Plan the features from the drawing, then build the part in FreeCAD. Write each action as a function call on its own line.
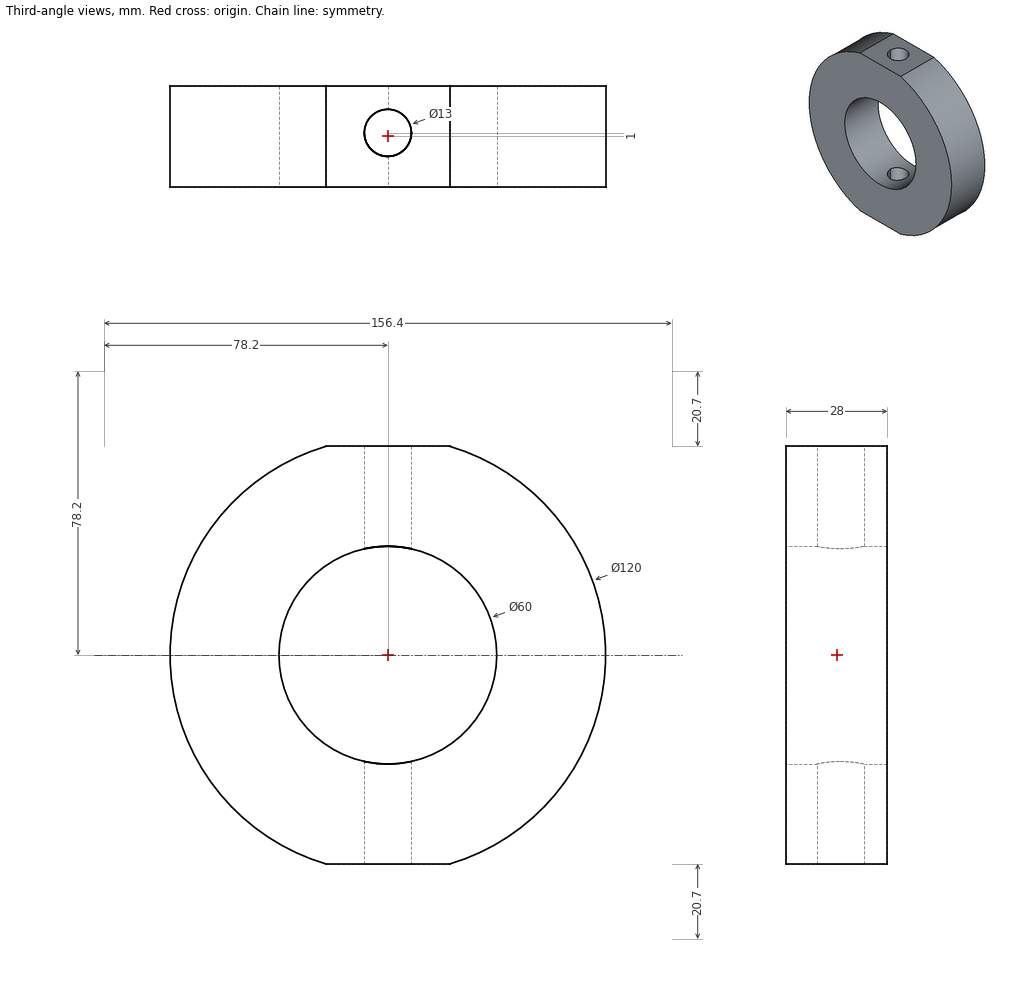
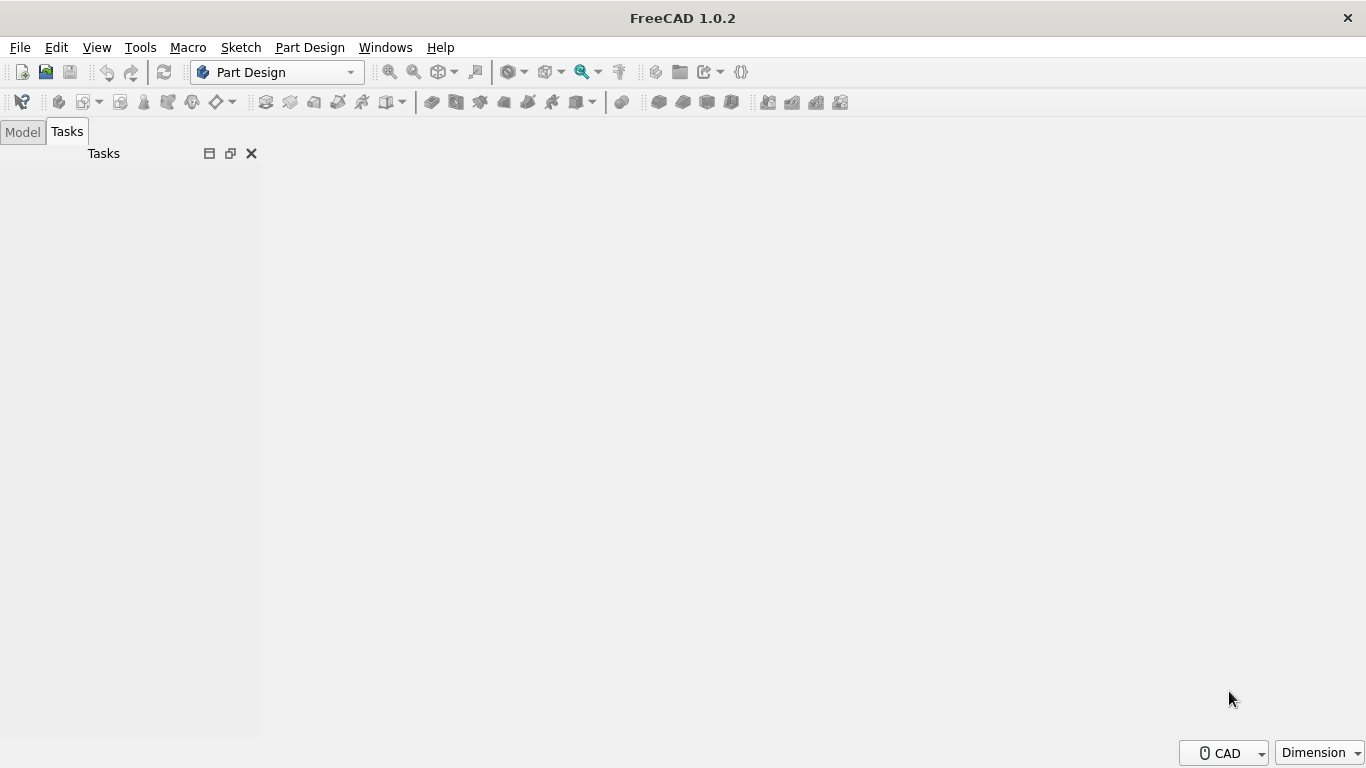
key(ctrl+n)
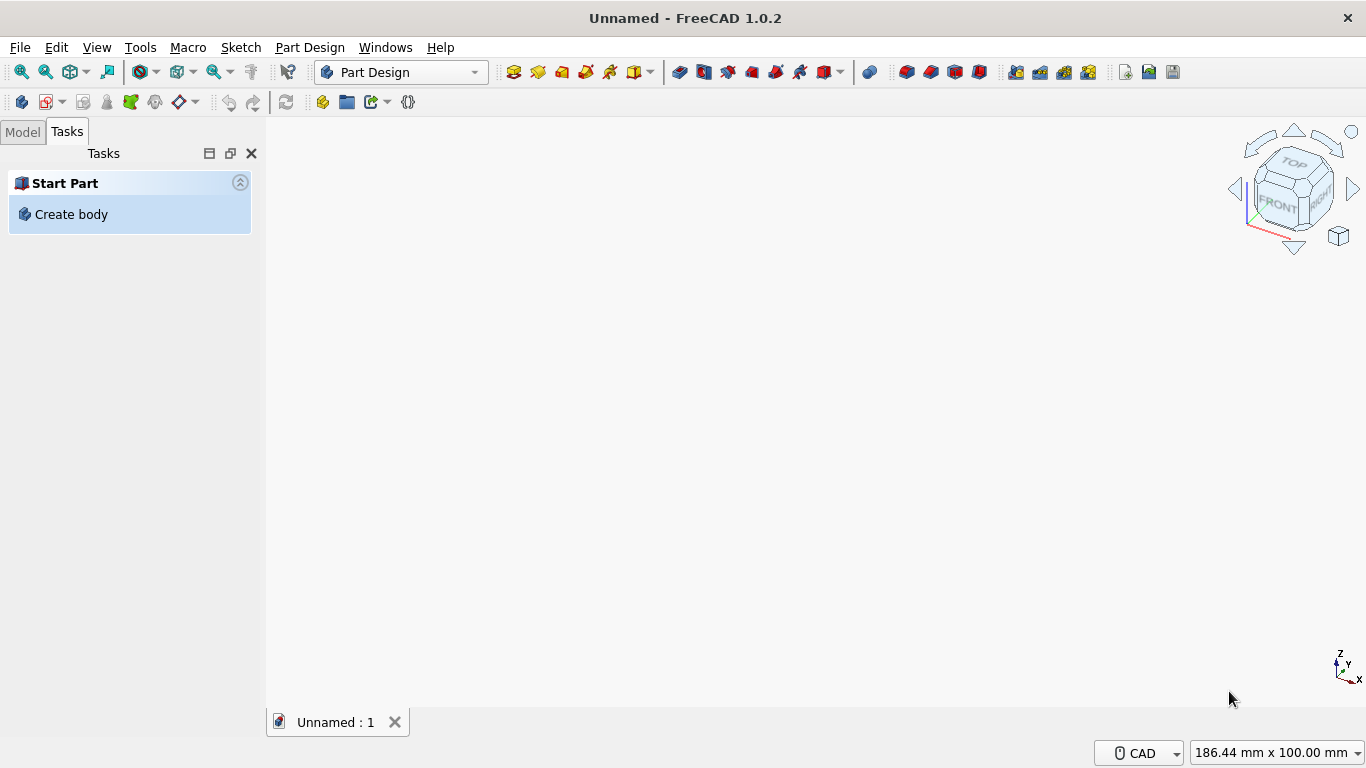
click(46, 102)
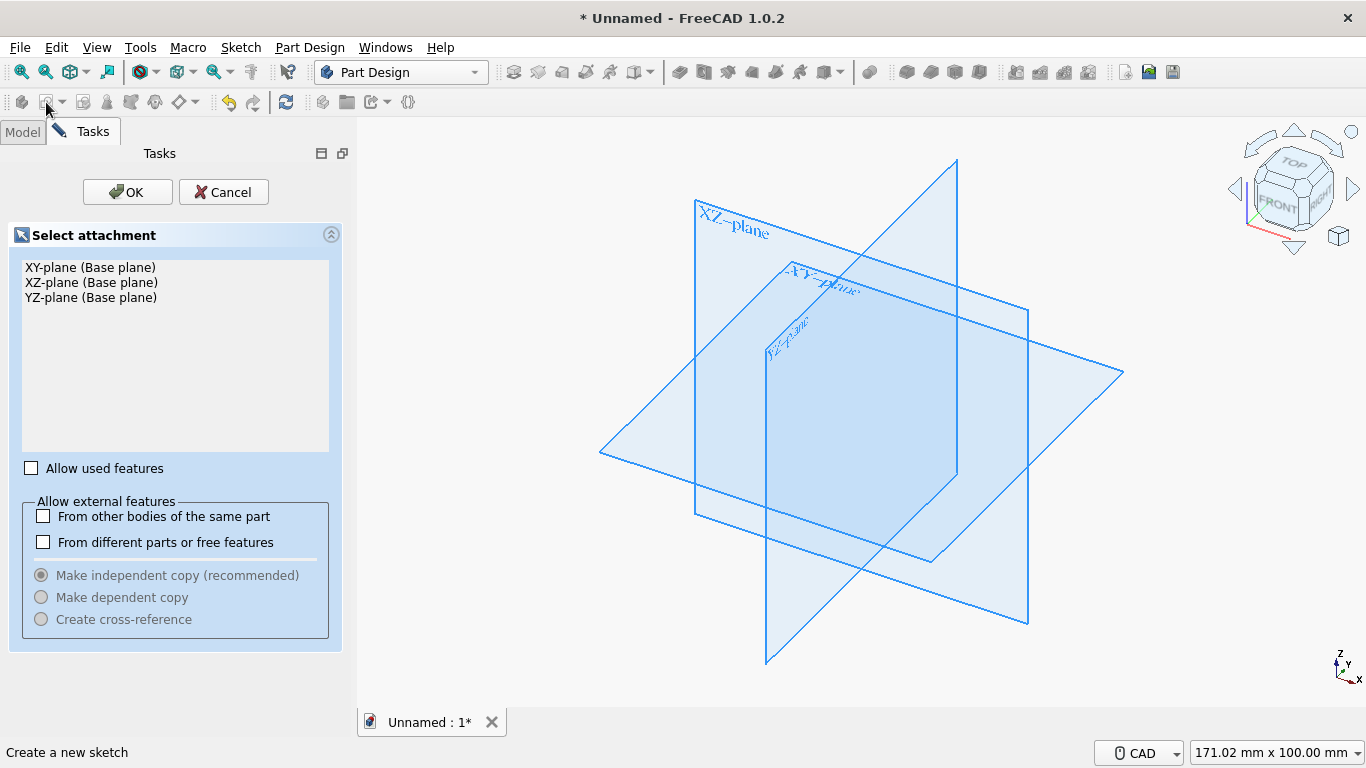
click(82, 282)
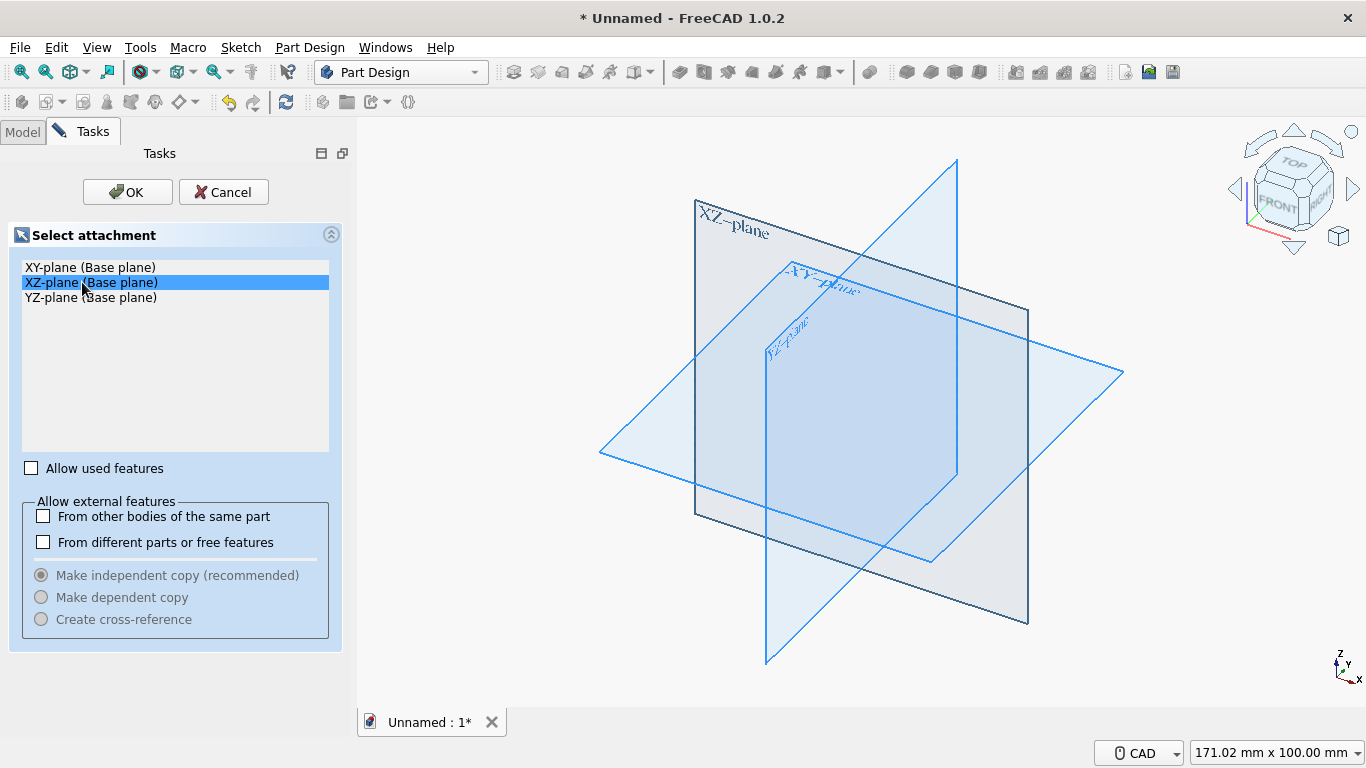
click(128, 192)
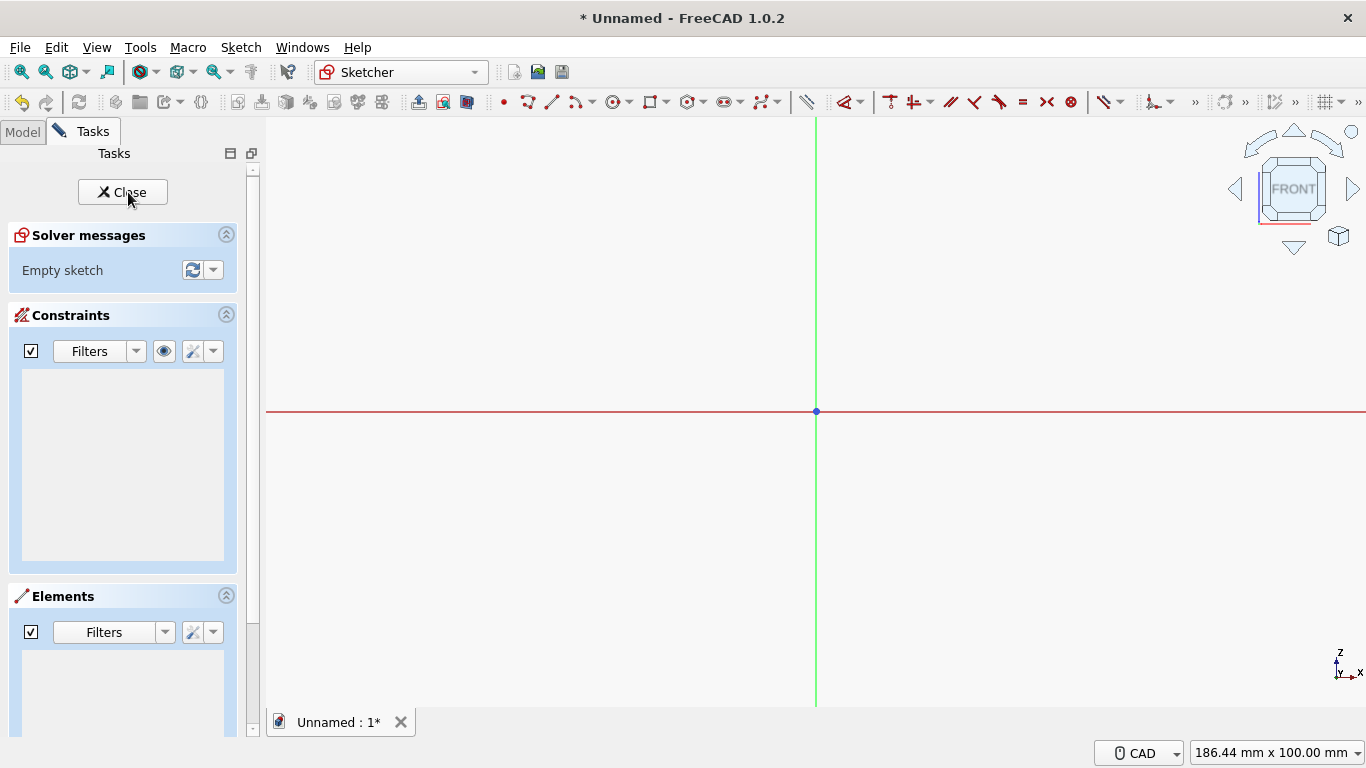
scroll(664, 412, down, 3)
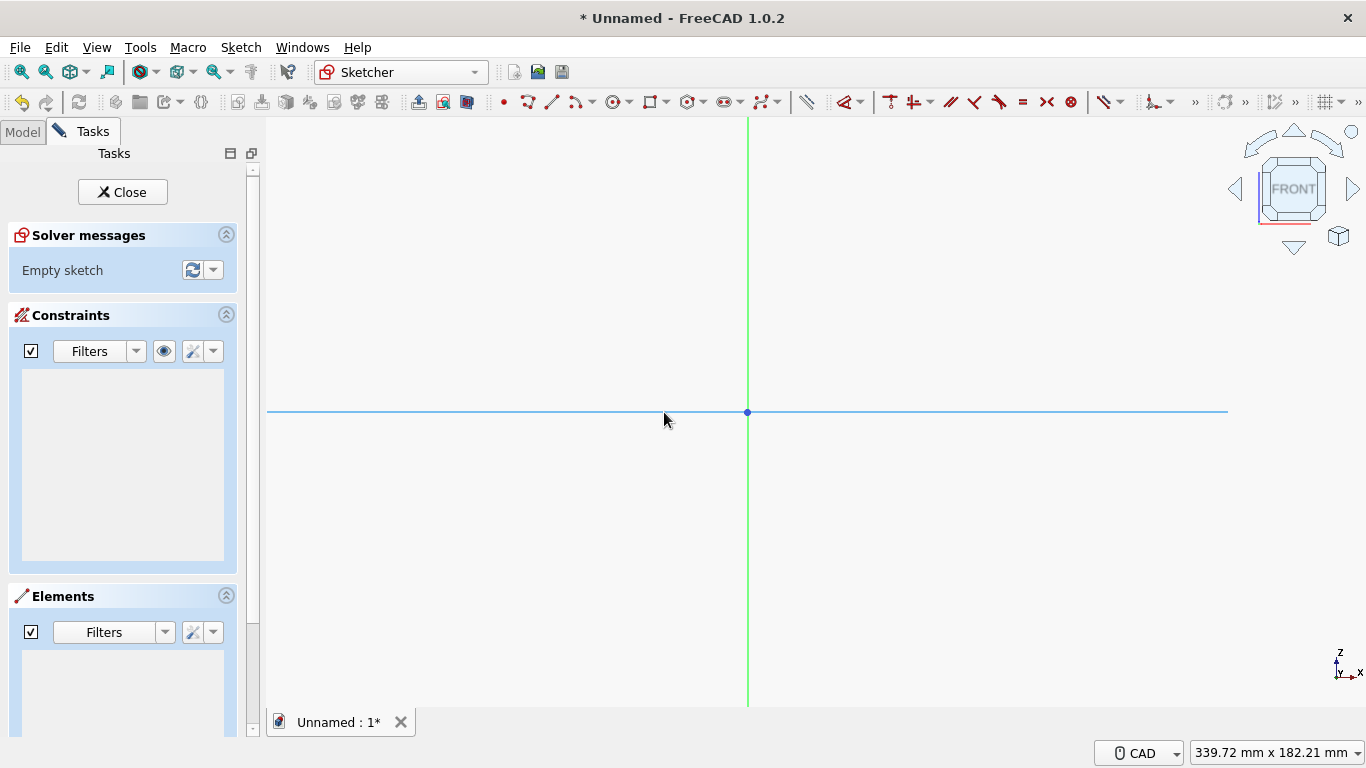
key(g)
key(c)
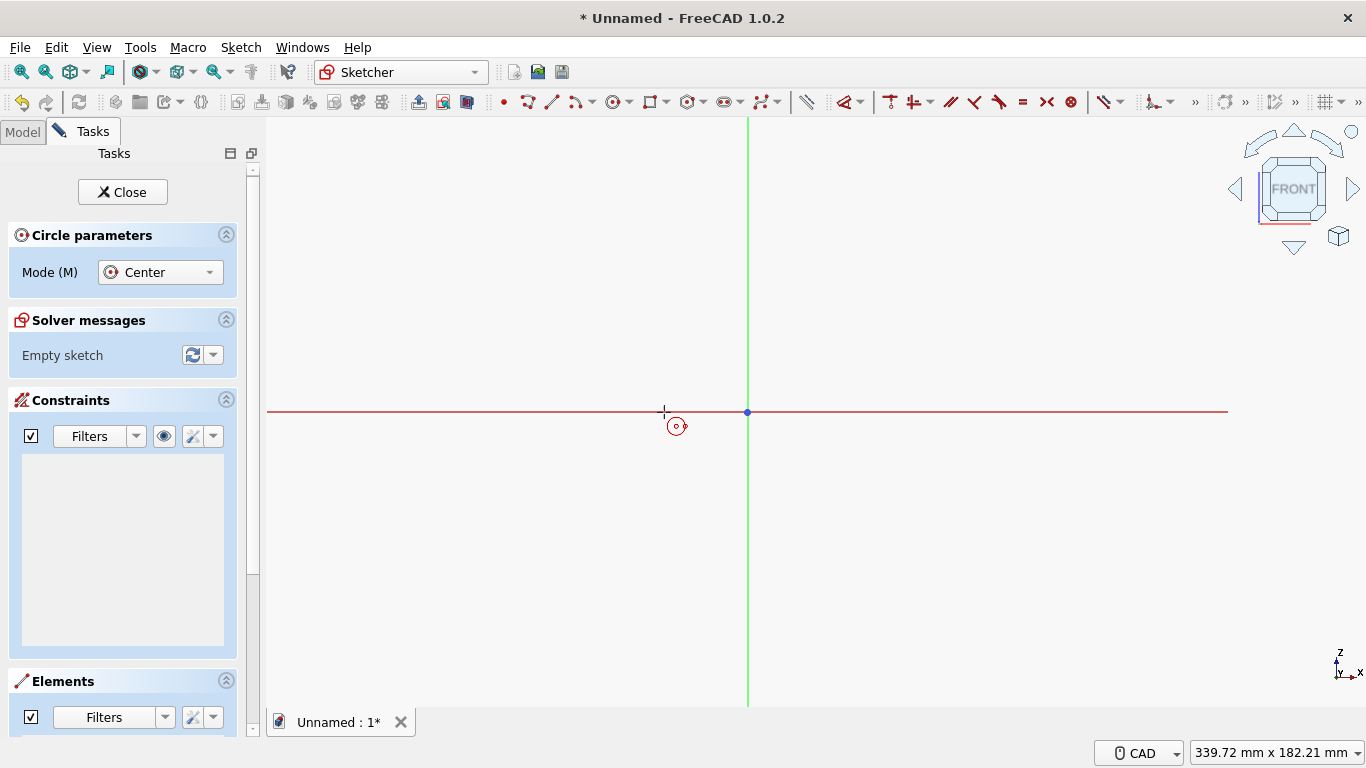
click(748, 412)
move(885, 275)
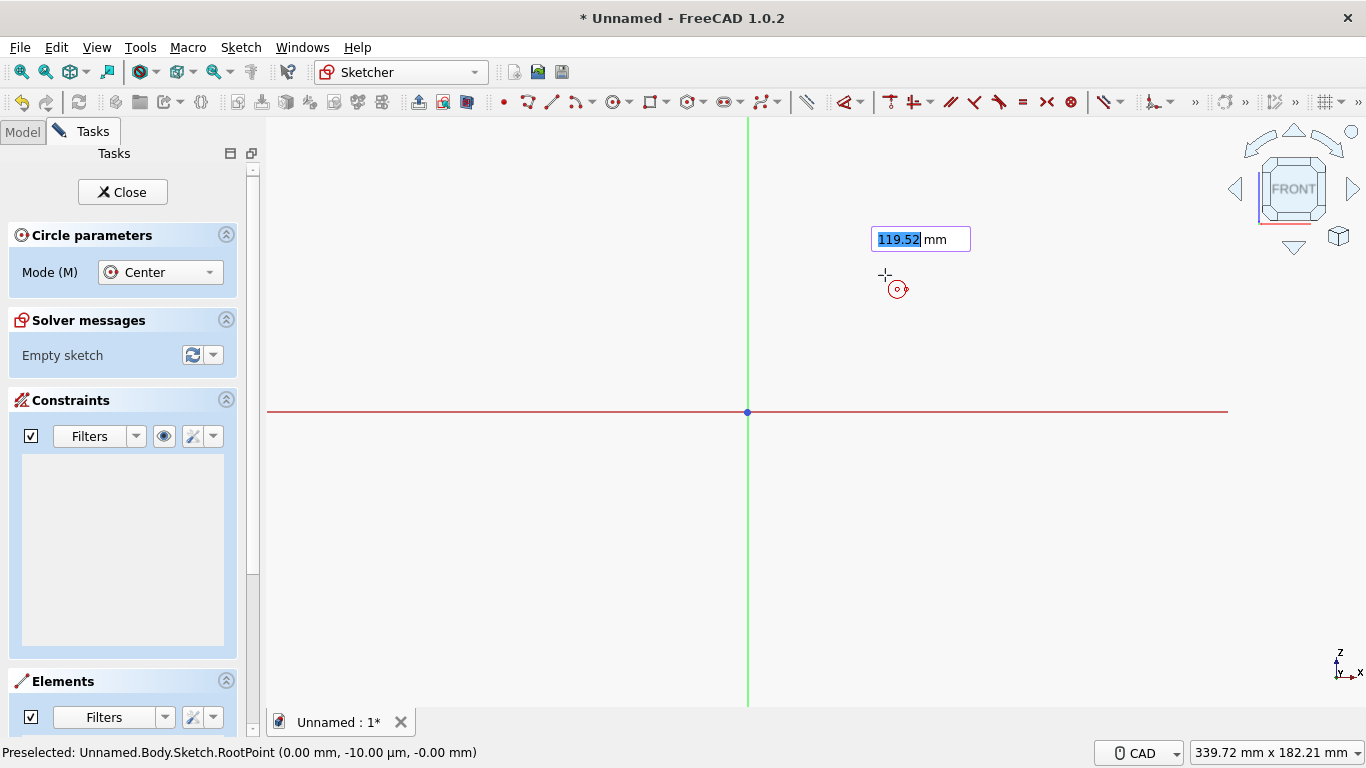
text(120)
key(Return)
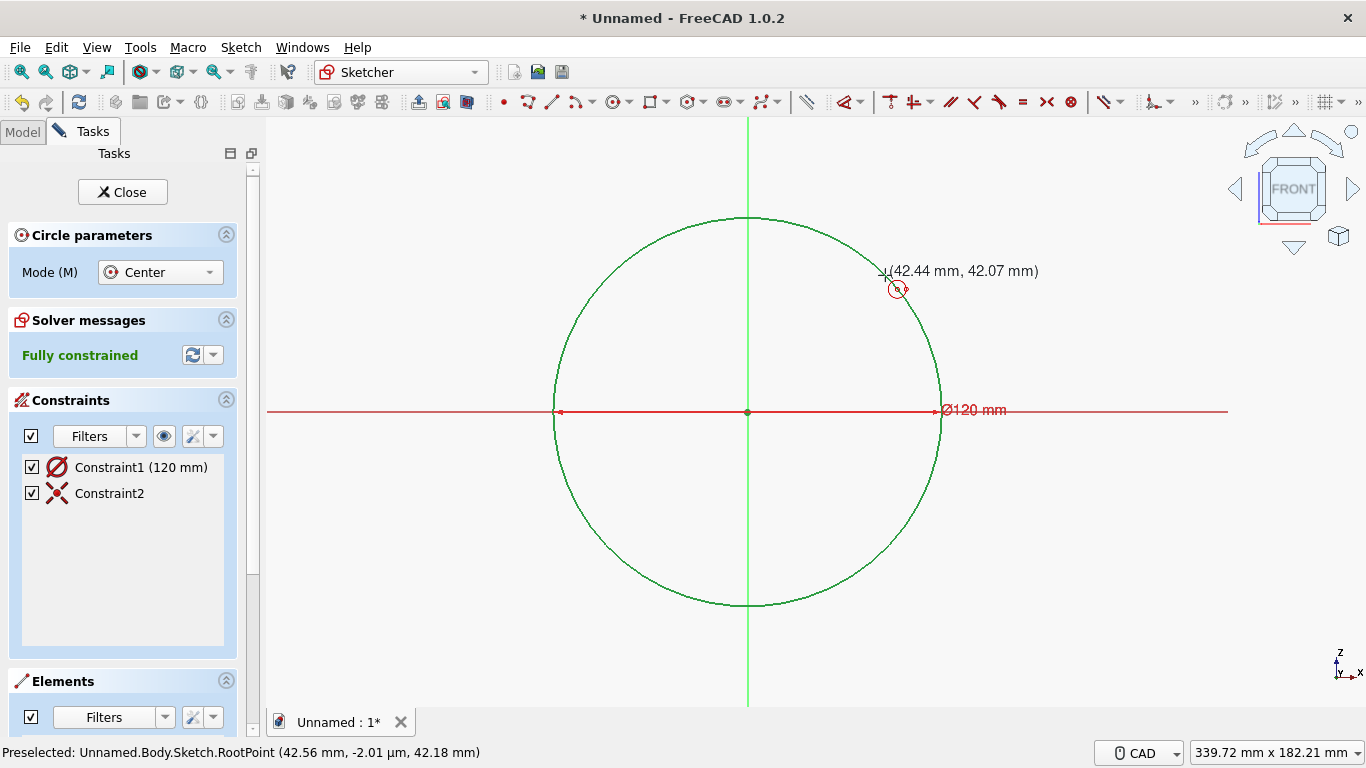
click(748, 412)
move(816, 344)